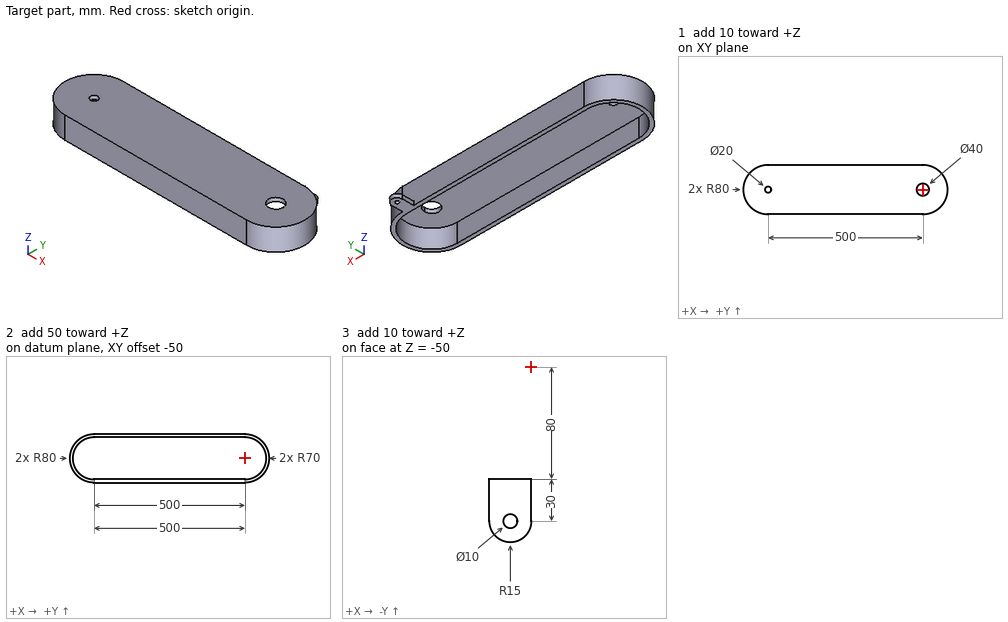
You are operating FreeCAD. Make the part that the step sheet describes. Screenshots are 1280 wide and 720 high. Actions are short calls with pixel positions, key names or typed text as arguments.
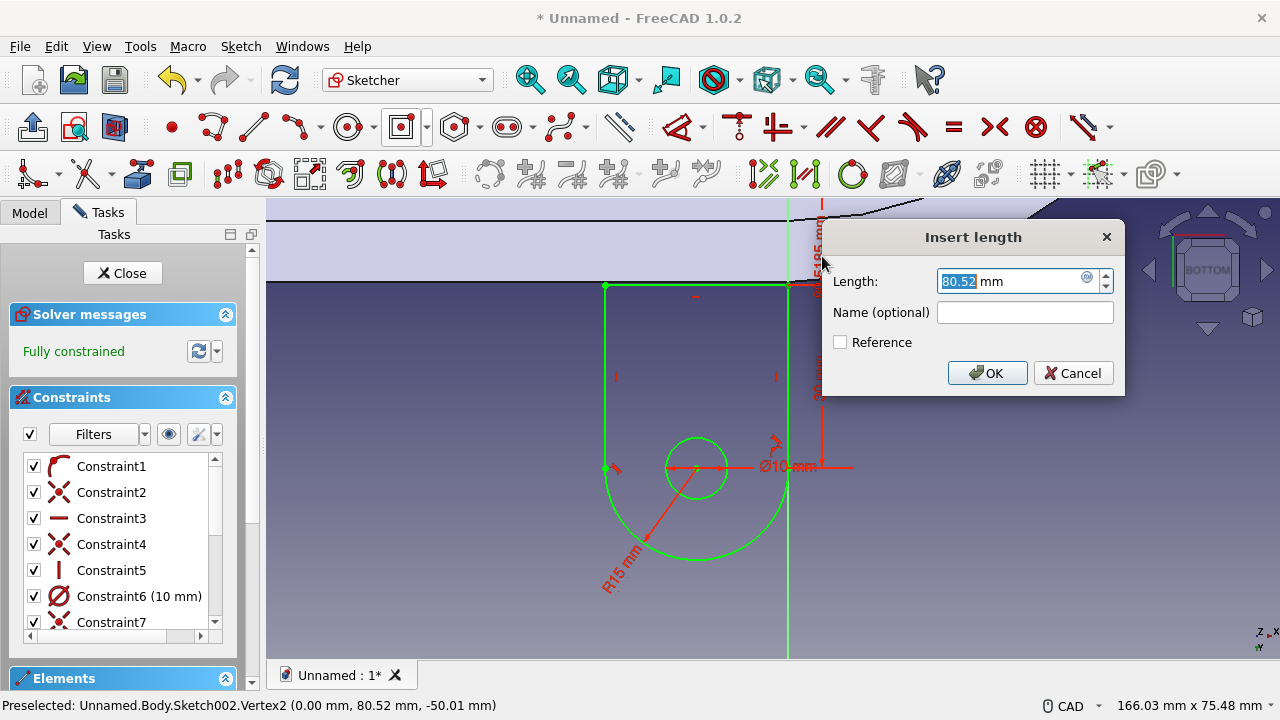
text(80)
key(Return)
key(Escape)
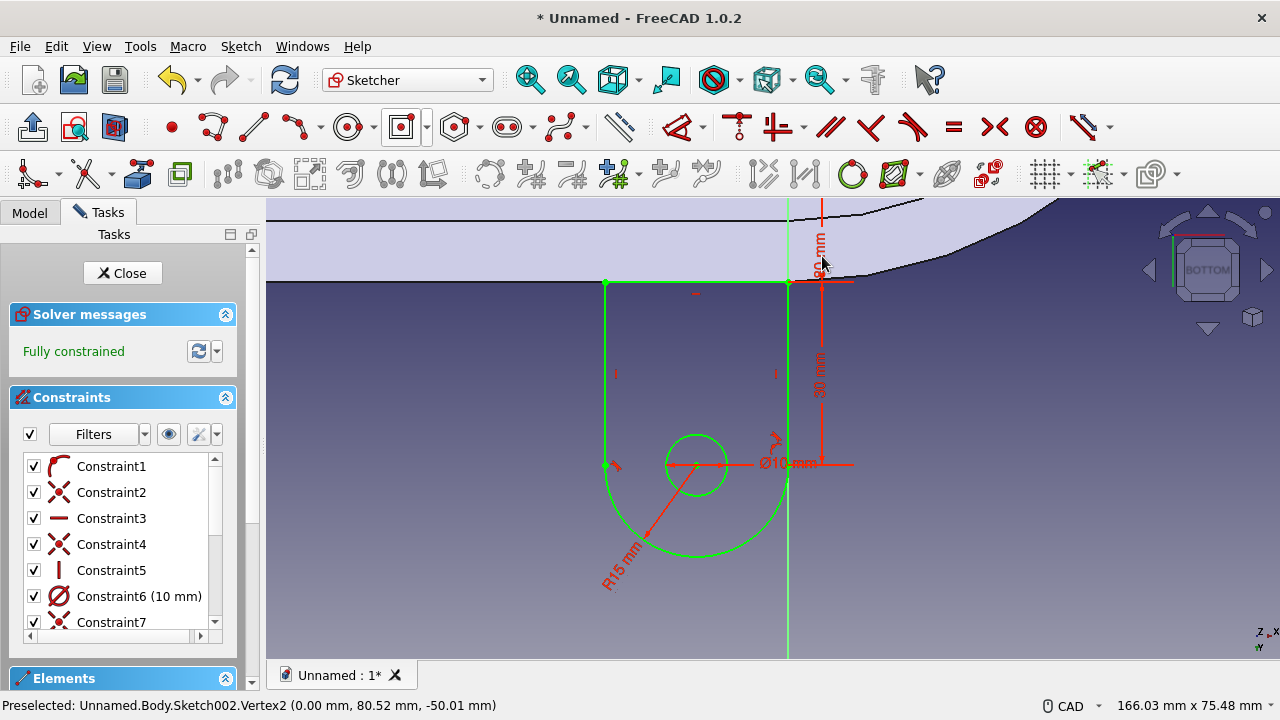
click(123, 273)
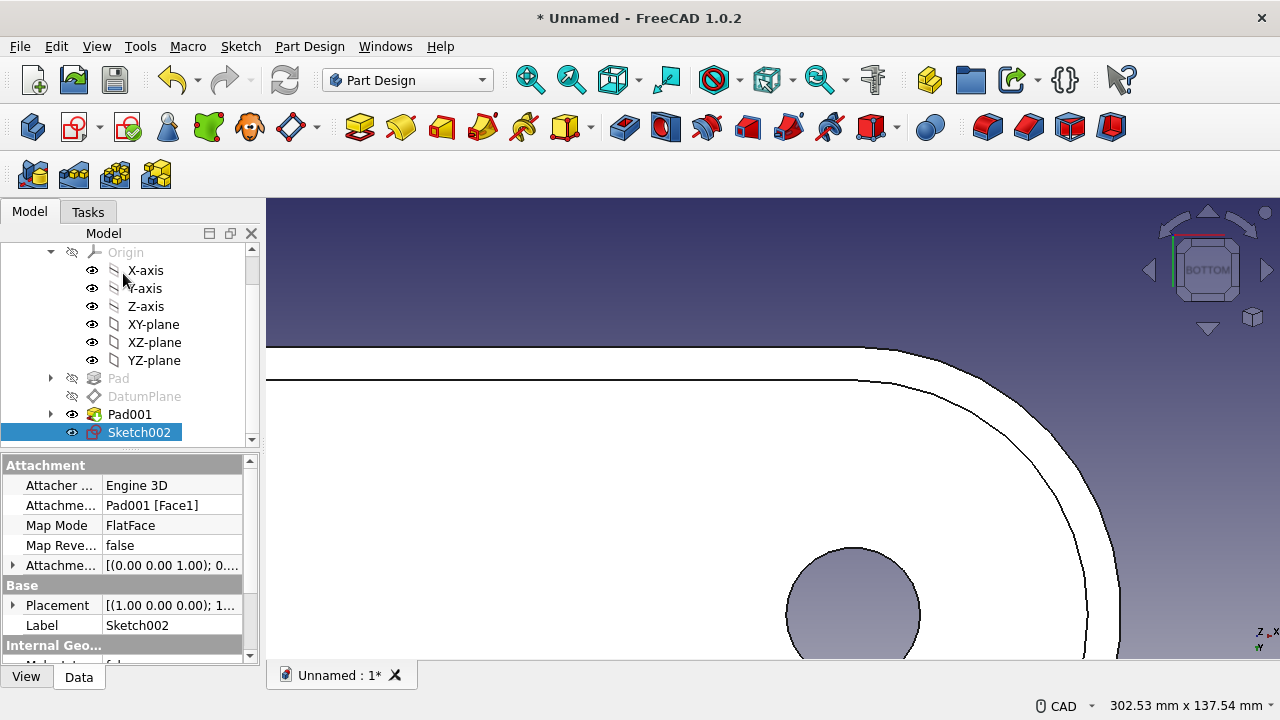
click(360, 128)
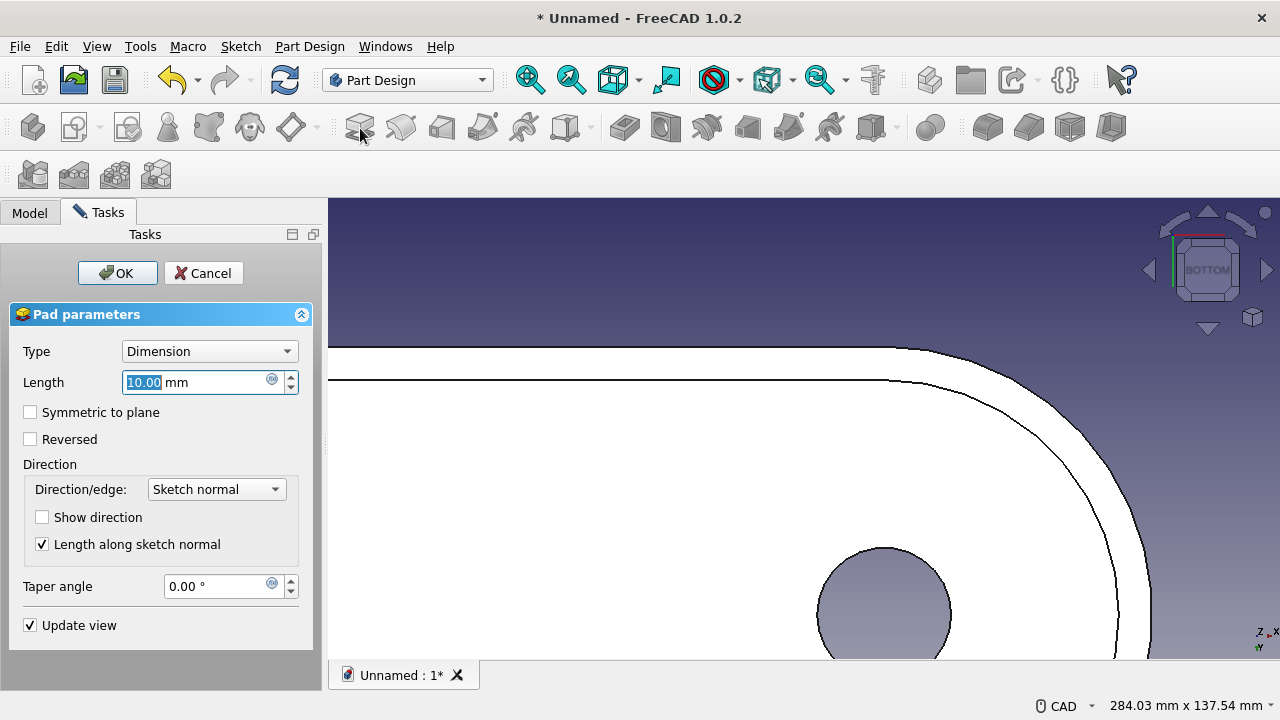
text(10)
key(Tab)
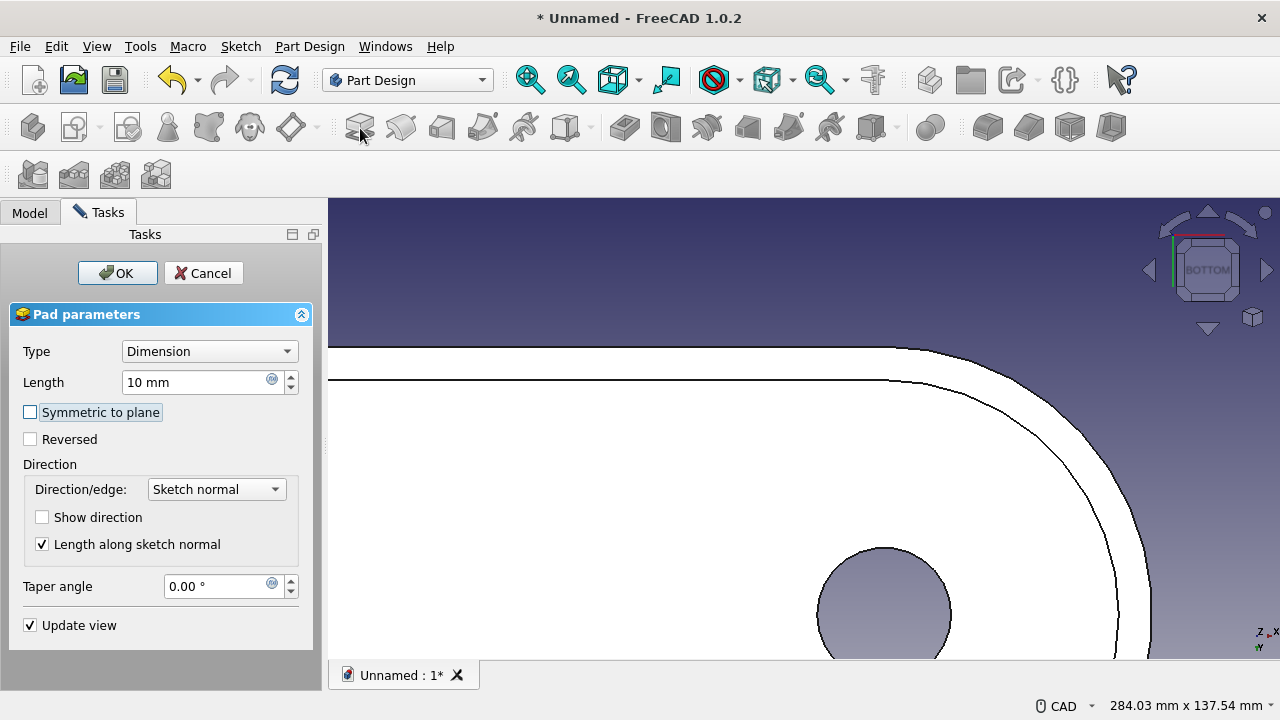
click(31, 439)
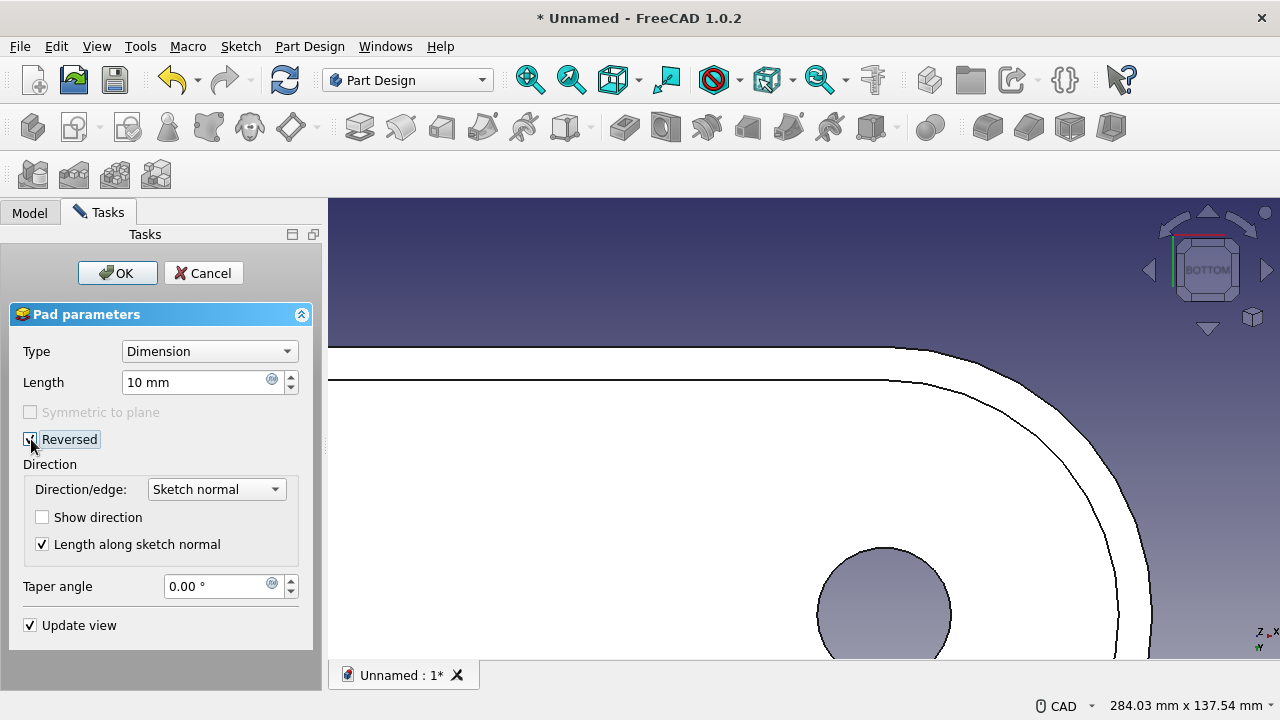
click(118, 273)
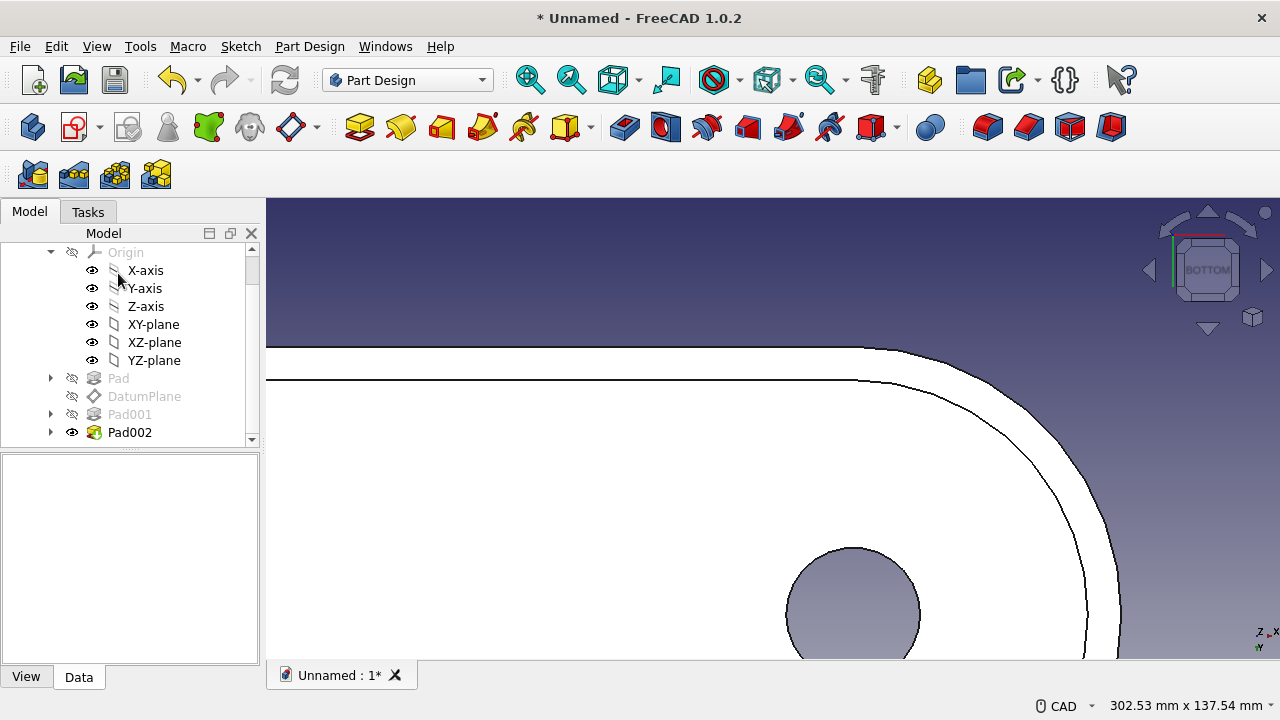
key(0)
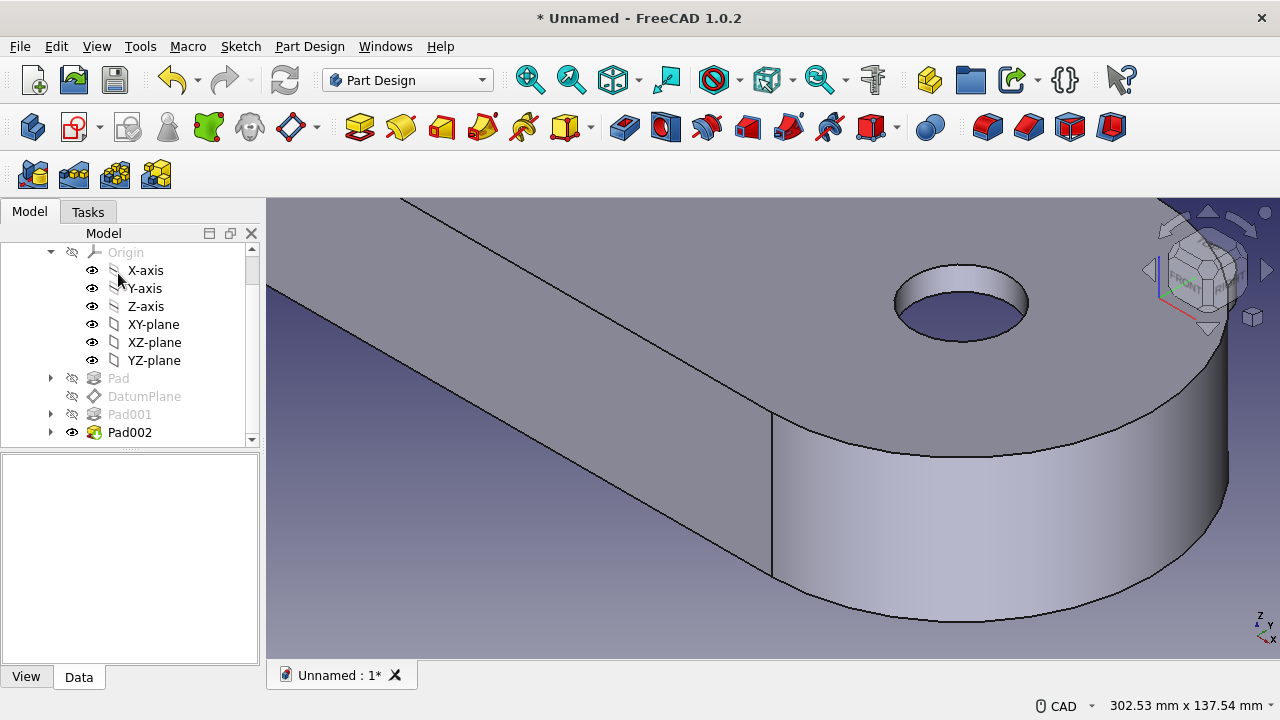
click(531, 80)